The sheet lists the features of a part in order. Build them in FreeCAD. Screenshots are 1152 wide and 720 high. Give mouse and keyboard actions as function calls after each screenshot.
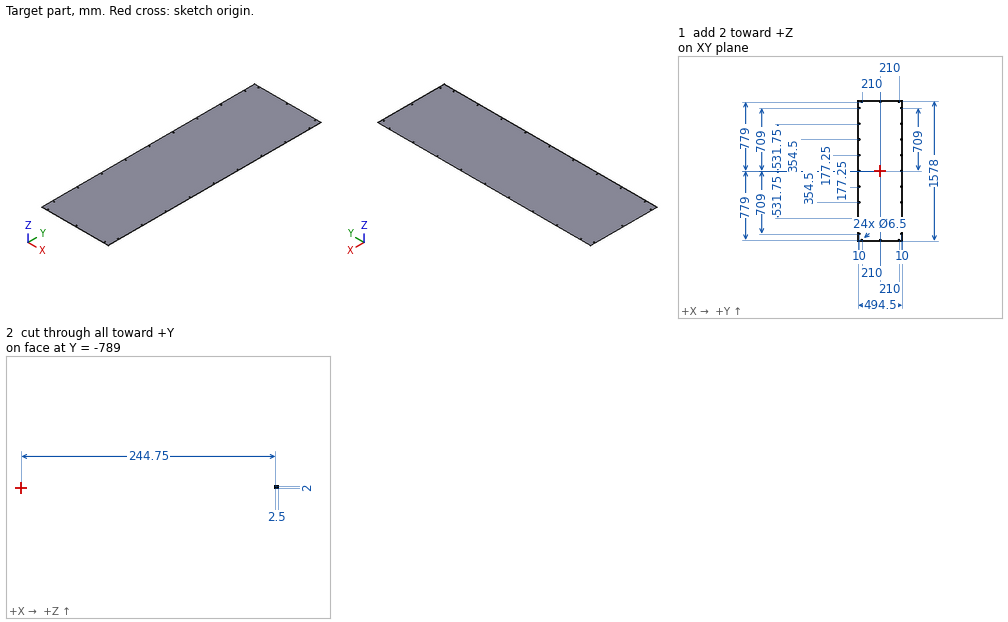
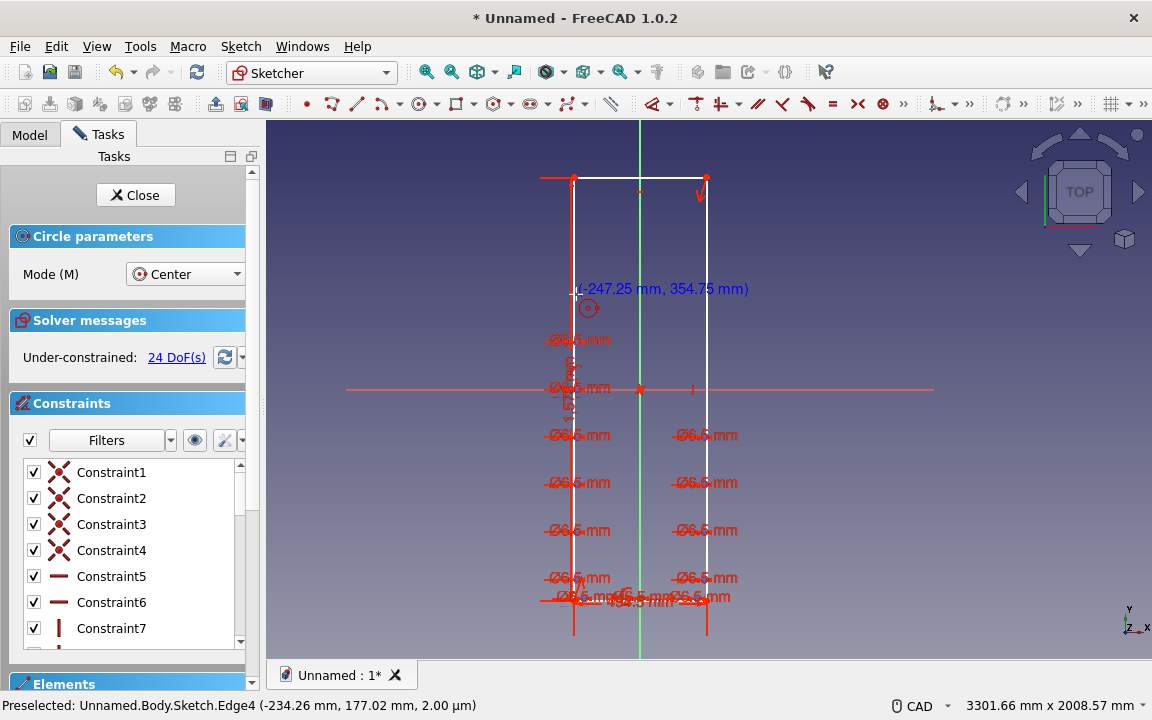
scroll(577, 294, up, 9)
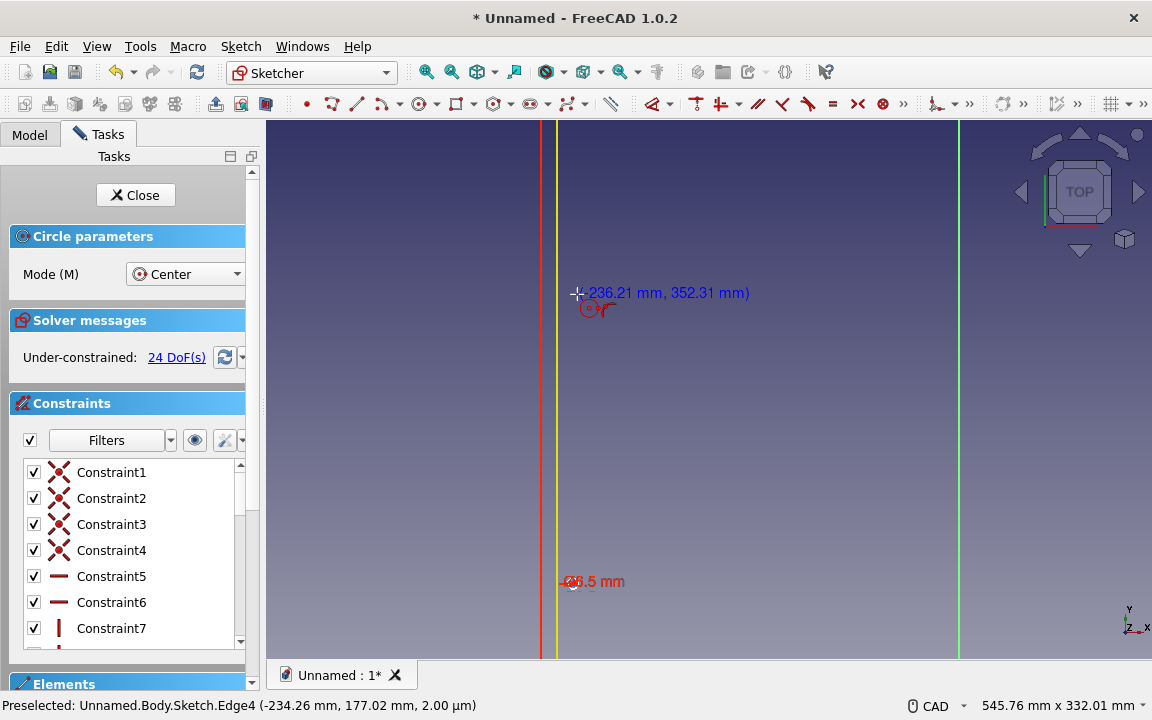
click(574, 295)
move(577, 291)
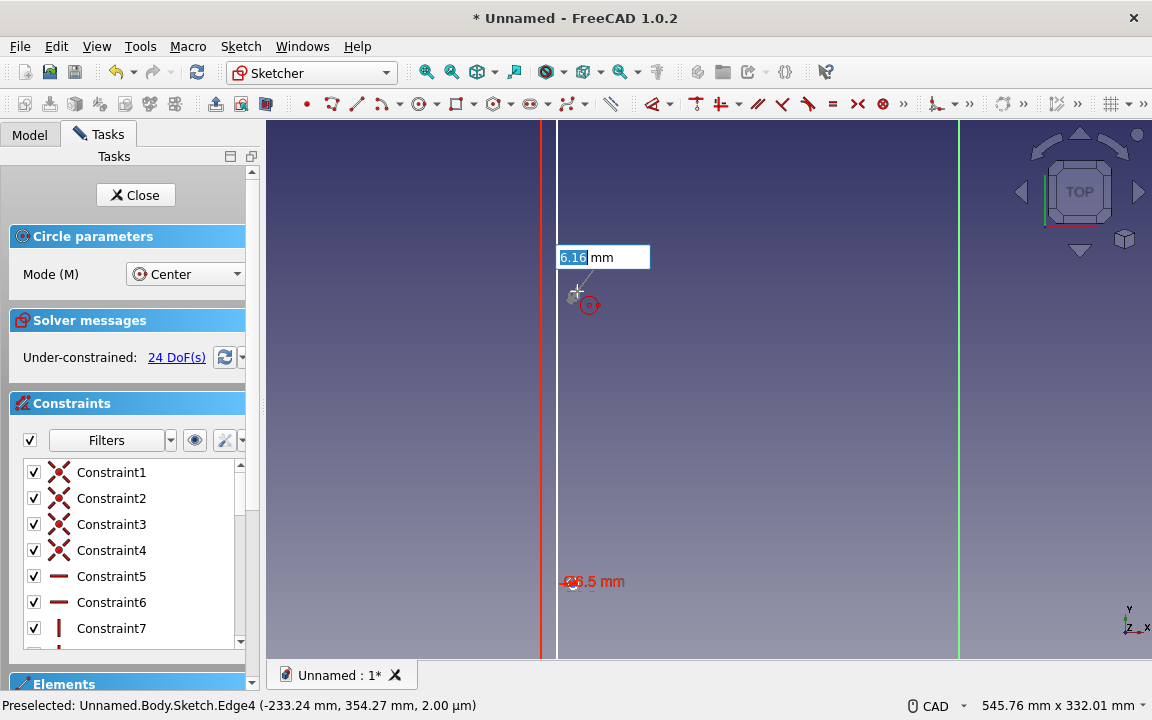
text(6.5)
key(Return)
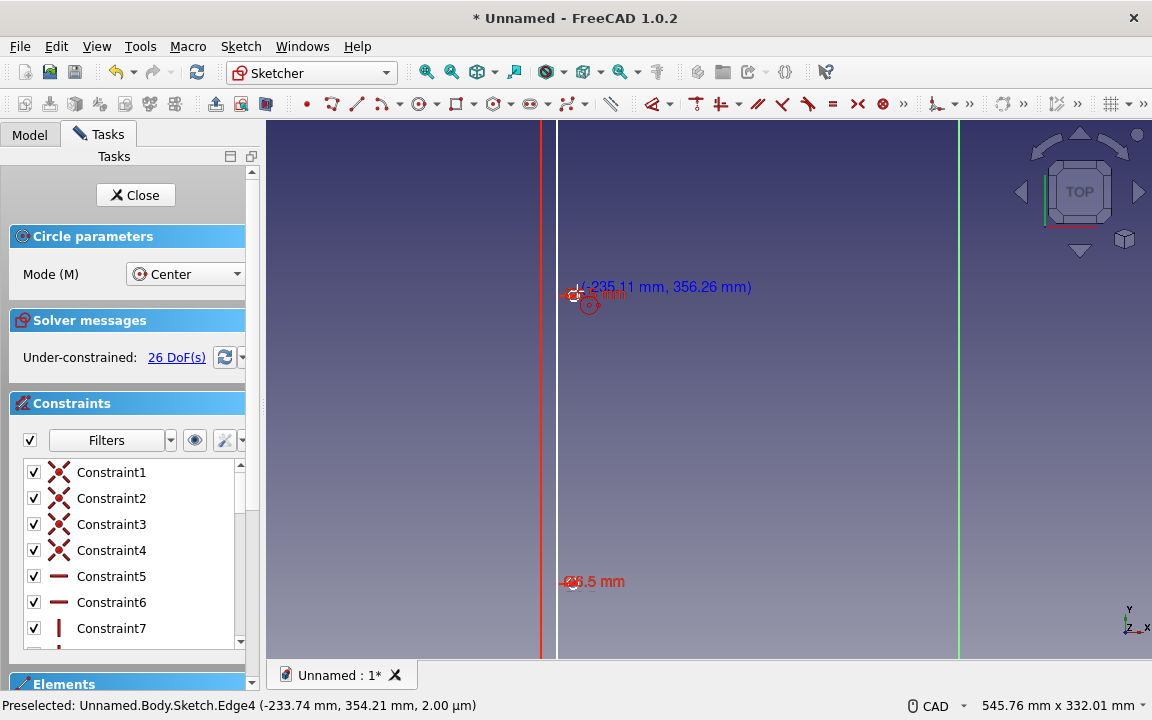
scroll(591, 314, down, 10)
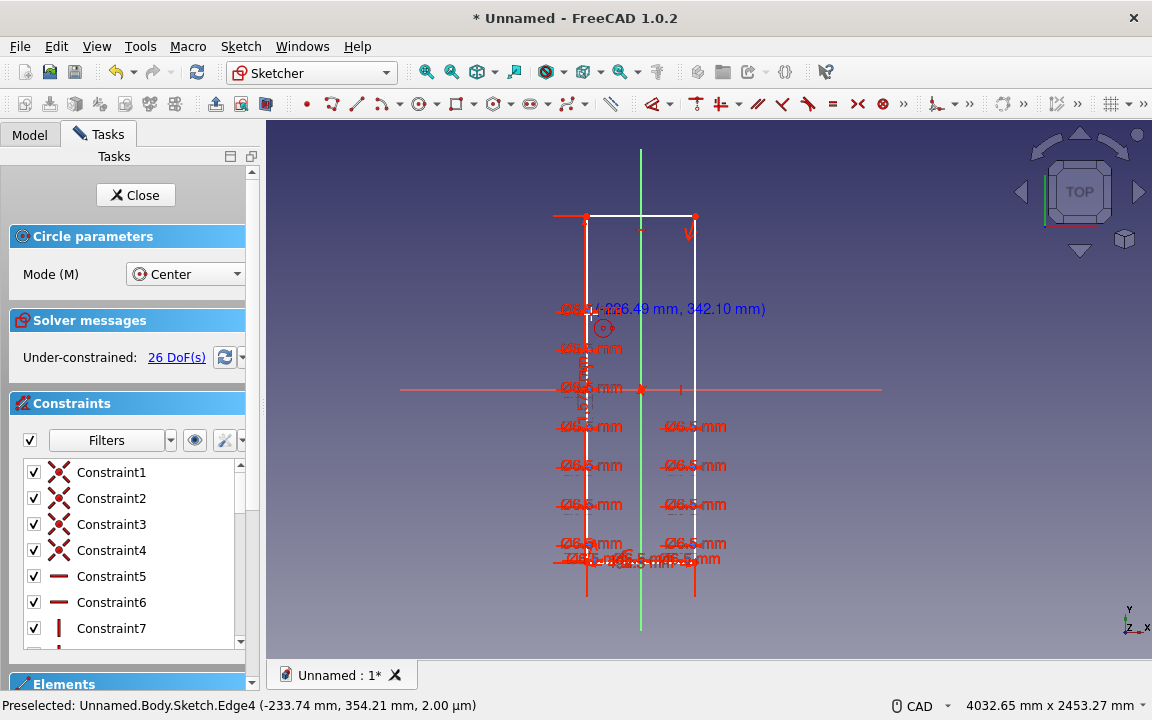
scroll(589, 273, up, 18)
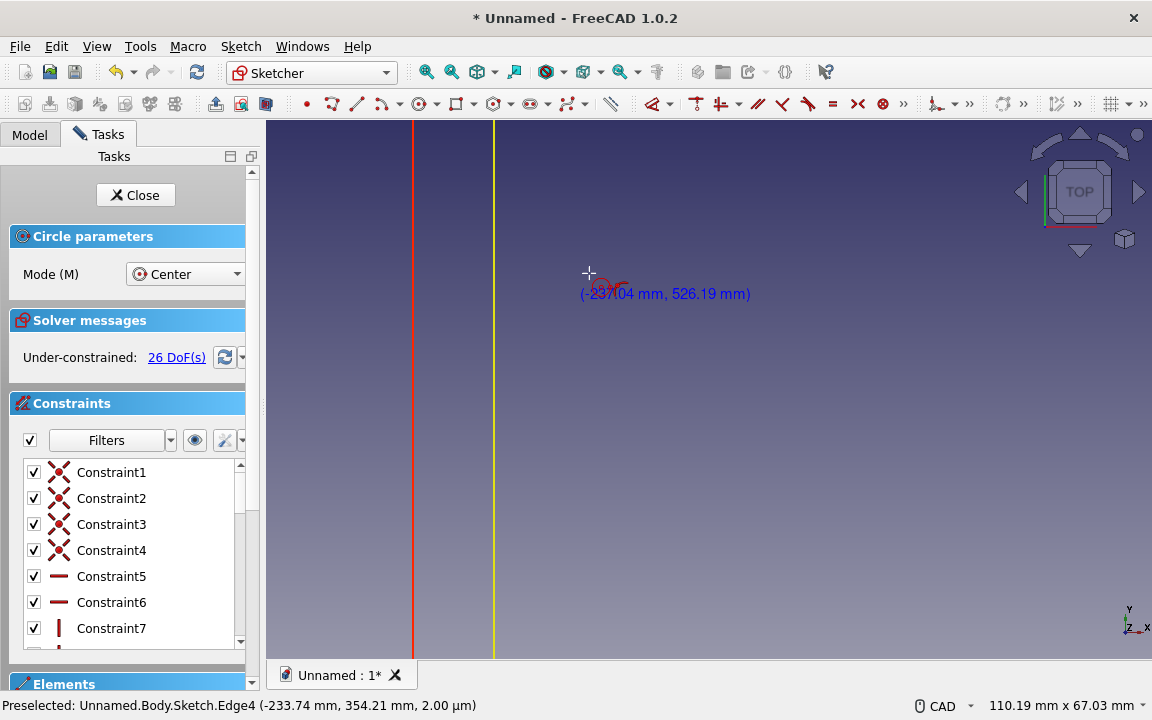
scroll(577, 247, down, 17)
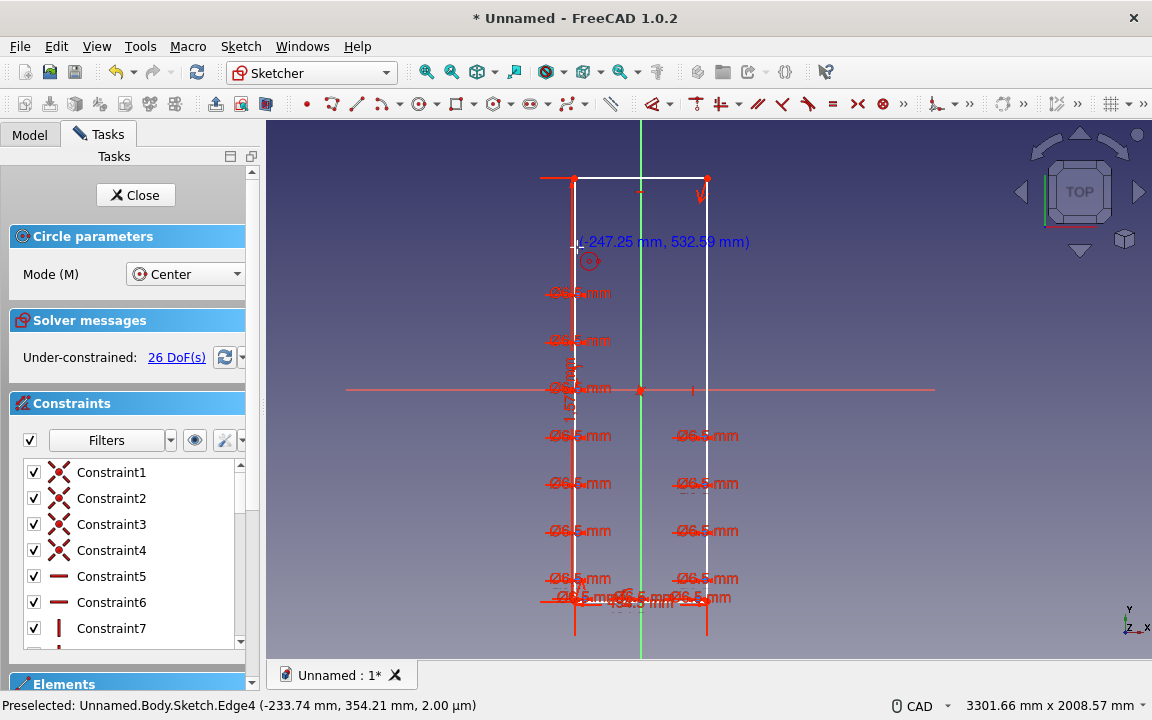
scroll(577, 247, up, 9)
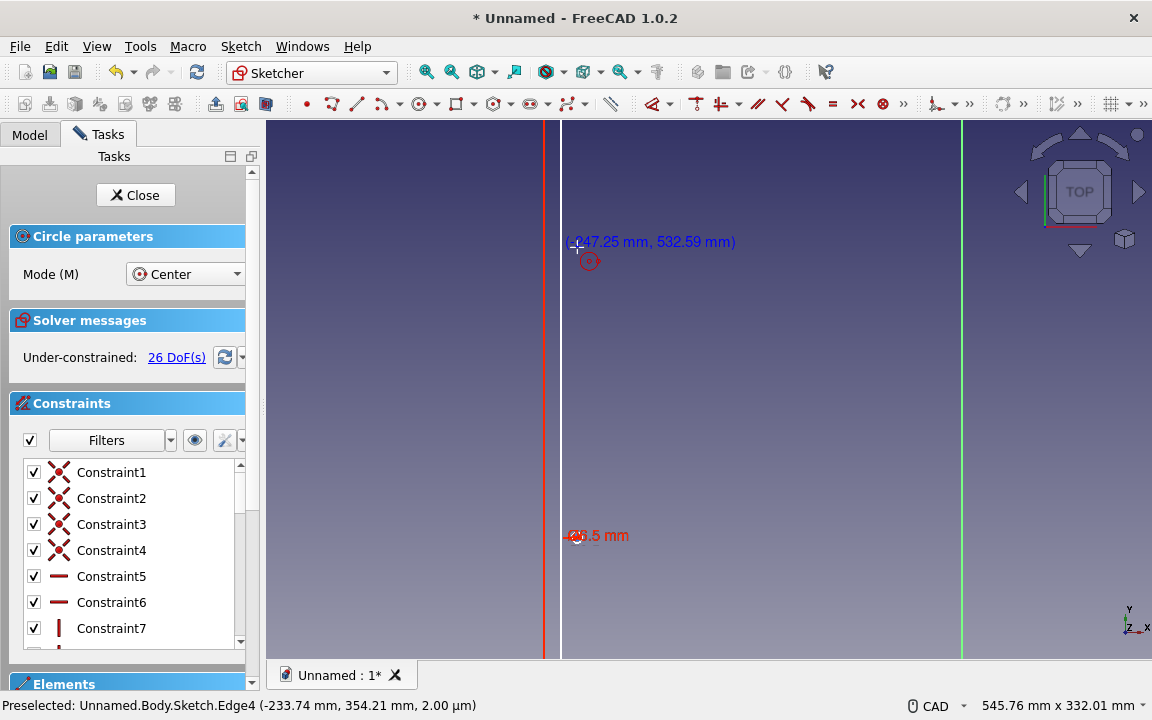
click(577, 249)
move(580, 245)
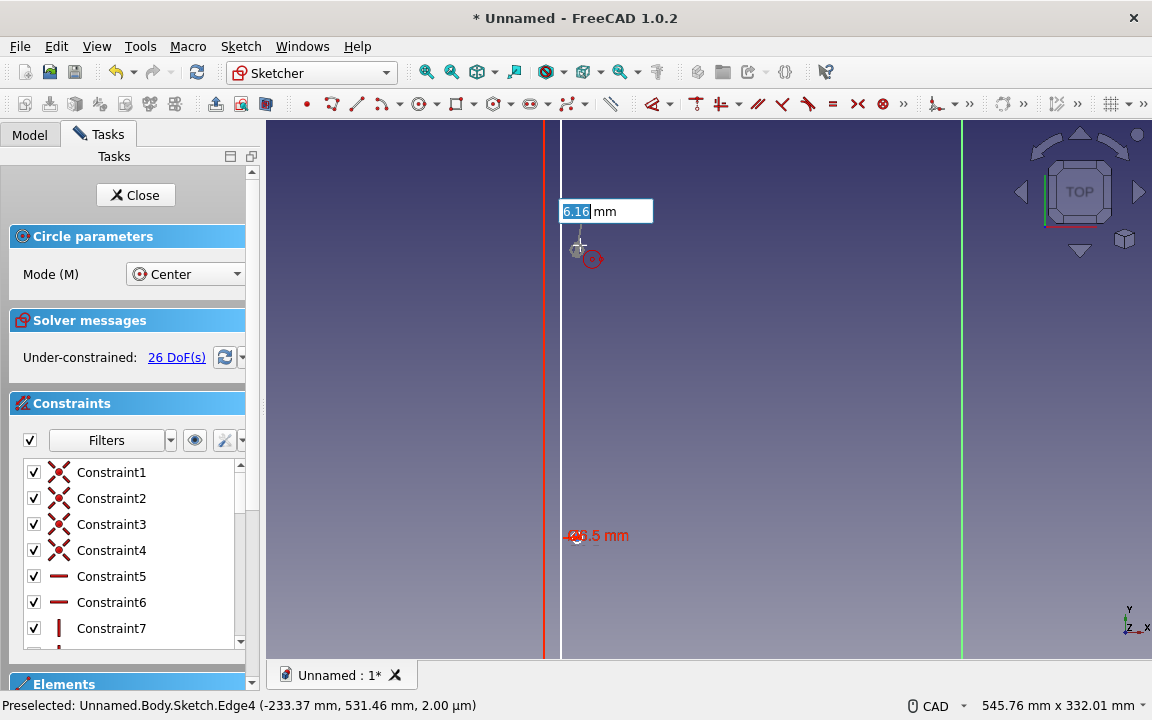
text(6.5)
key(Return)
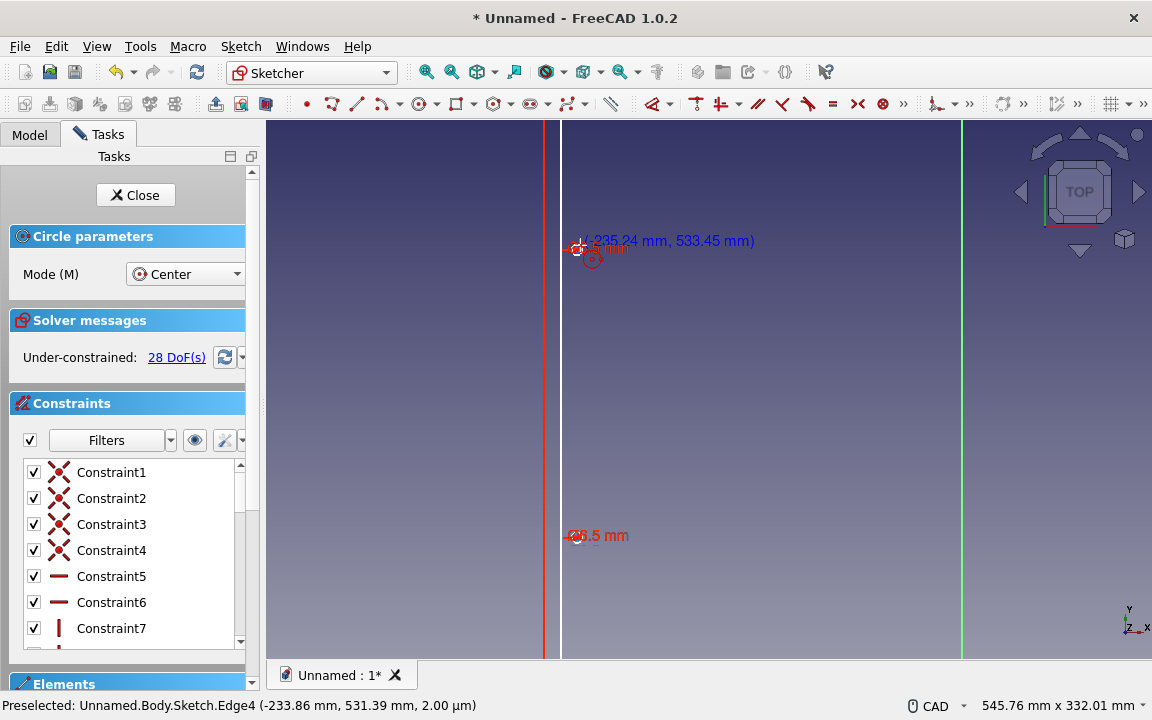
scroll(590, 276, down, 10)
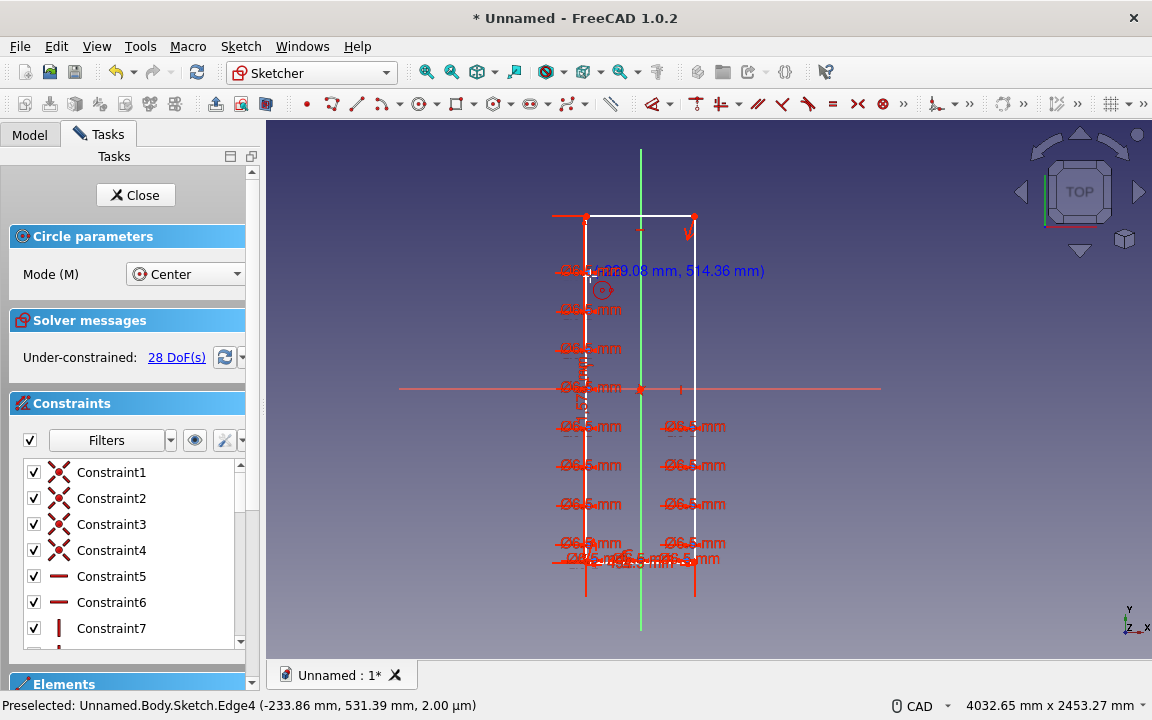
scroll(589, 234, up, 18)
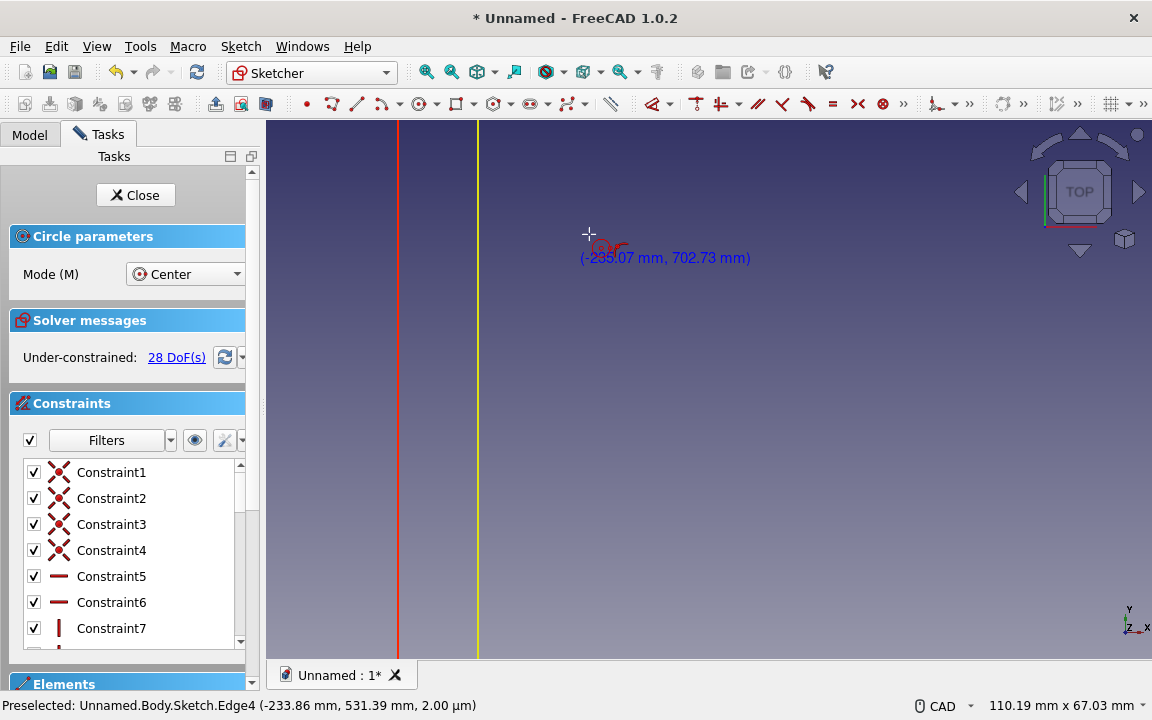
scroll(577, 199, down, 17)